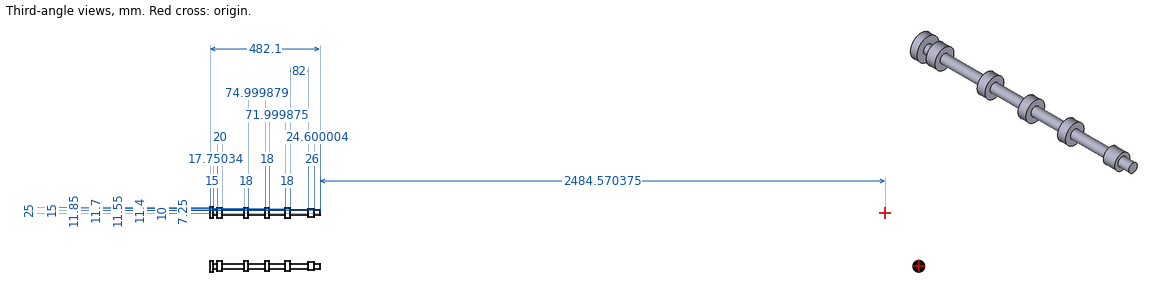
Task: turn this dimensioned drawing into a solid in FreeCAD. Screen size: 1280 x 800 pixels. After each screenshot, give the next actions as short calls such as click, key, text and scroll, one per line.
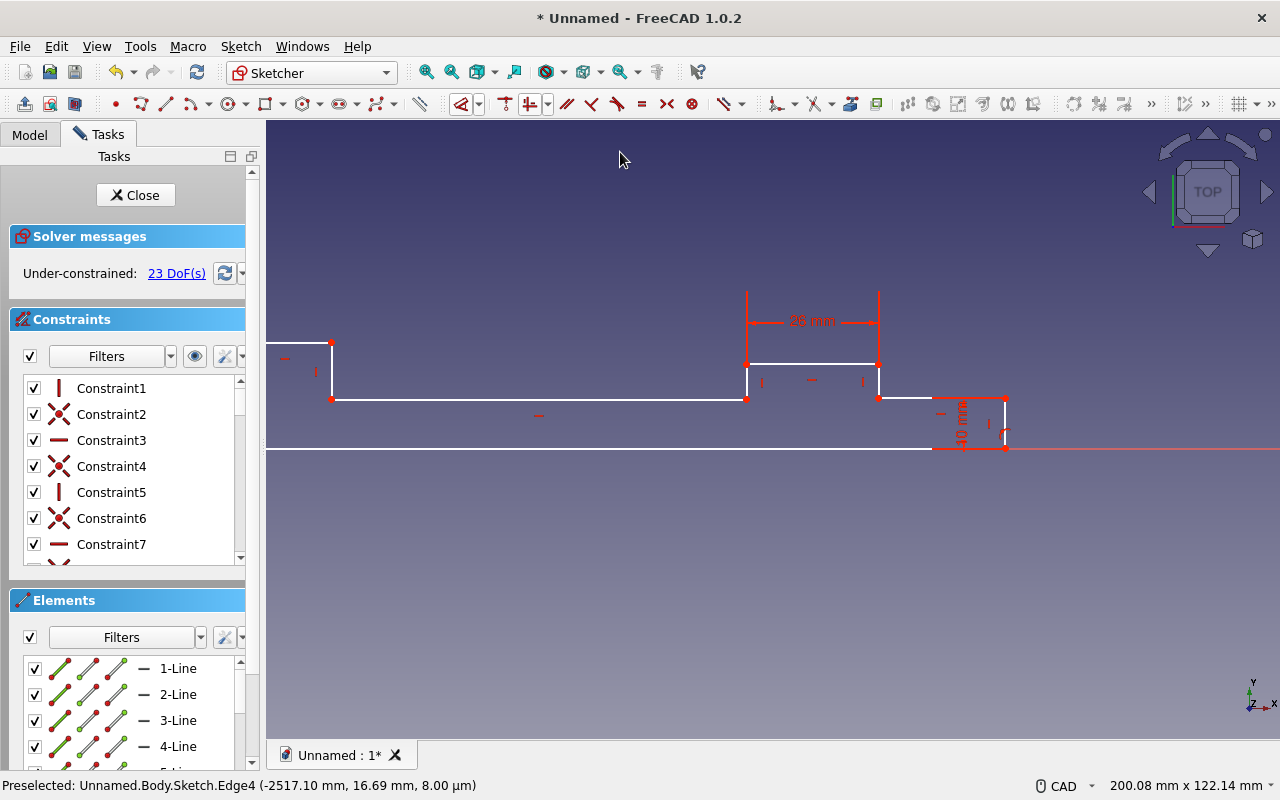
scroll(1006, 444, down, 7)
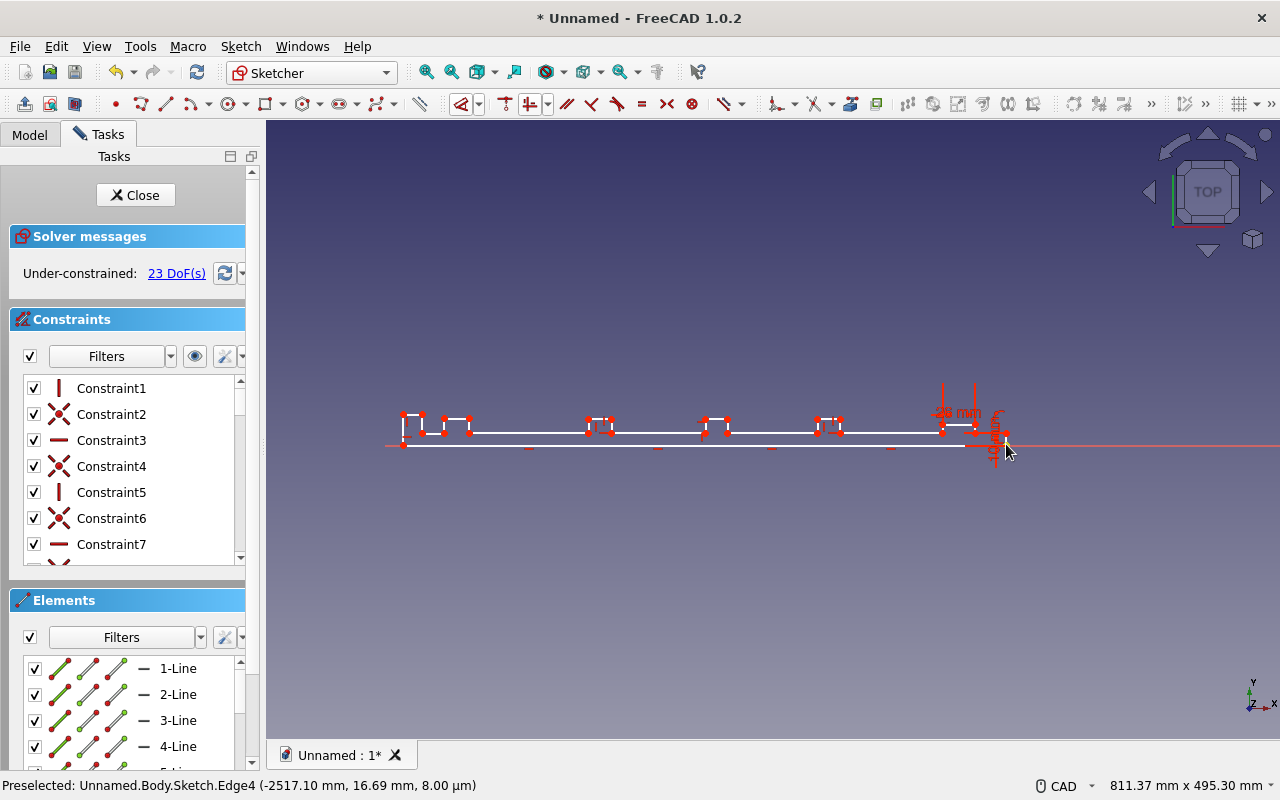
click(912, 433)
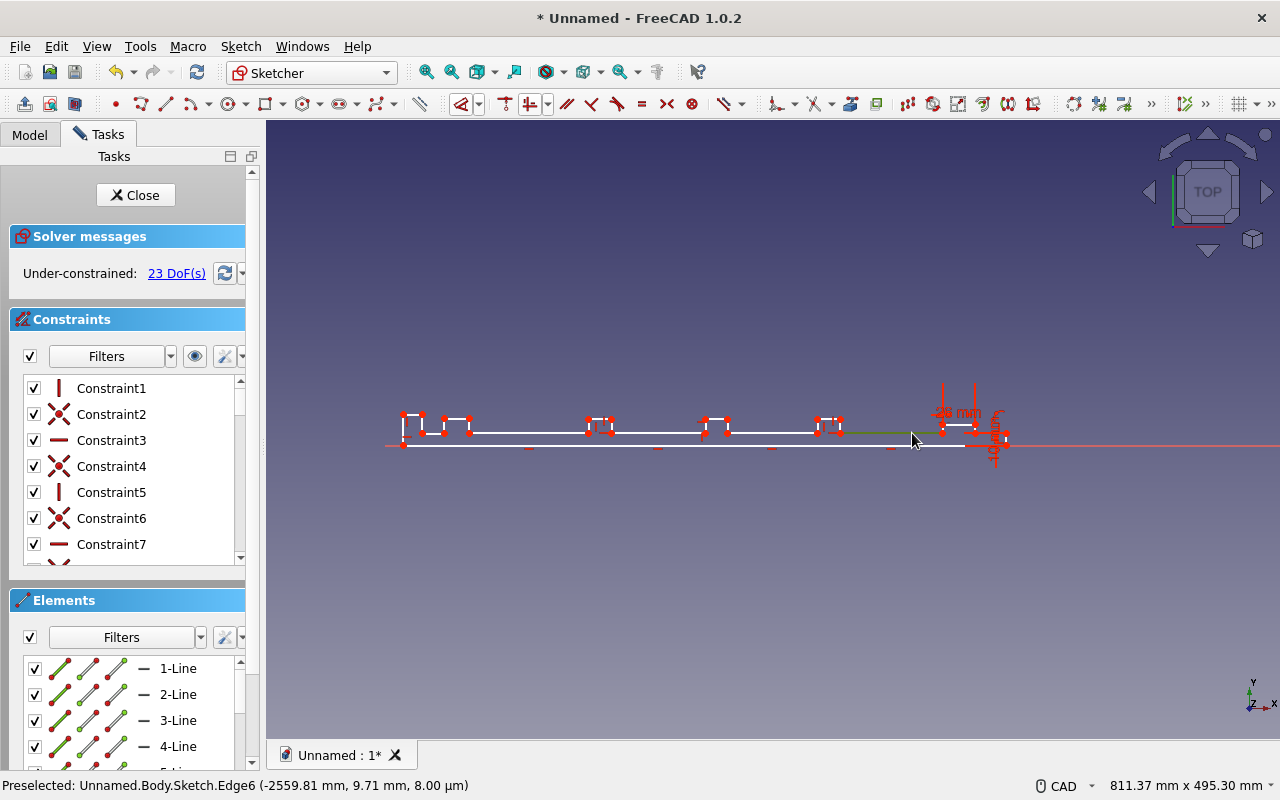
click(478, 104)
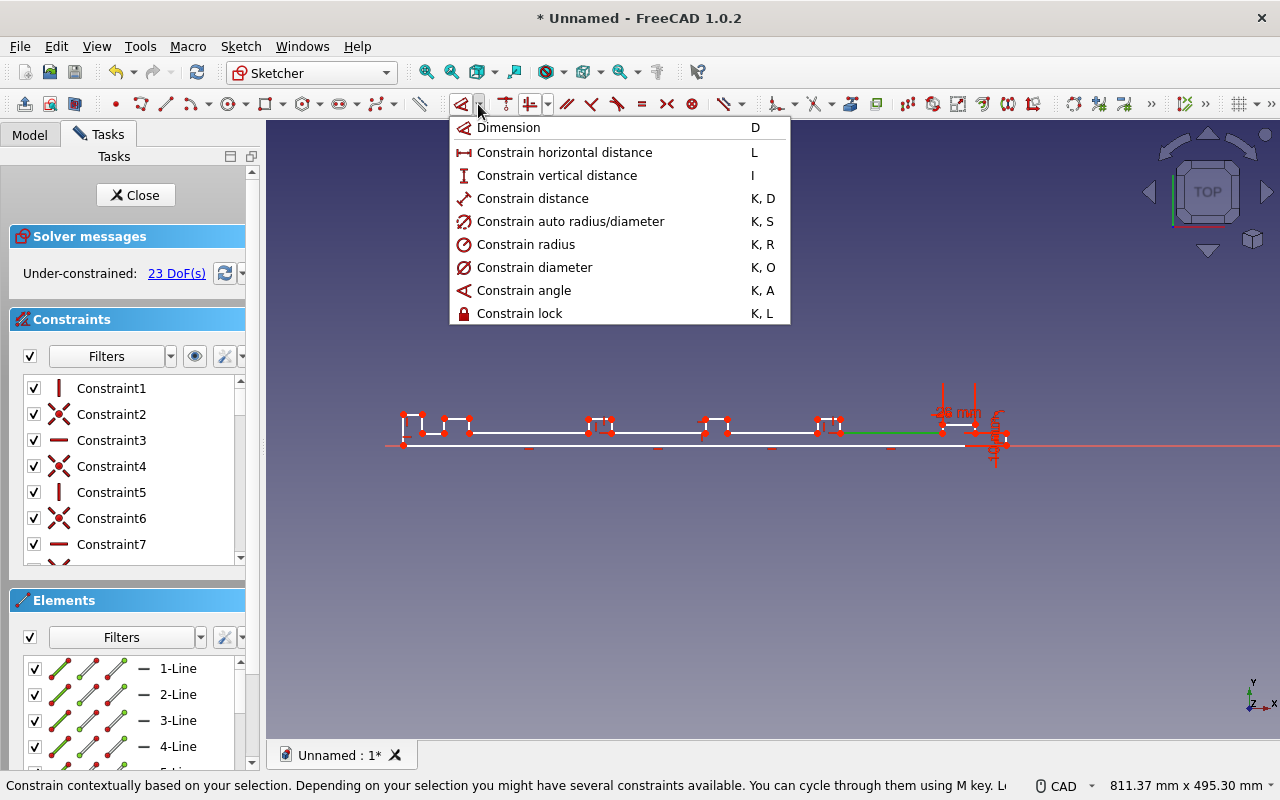
click(620, 152)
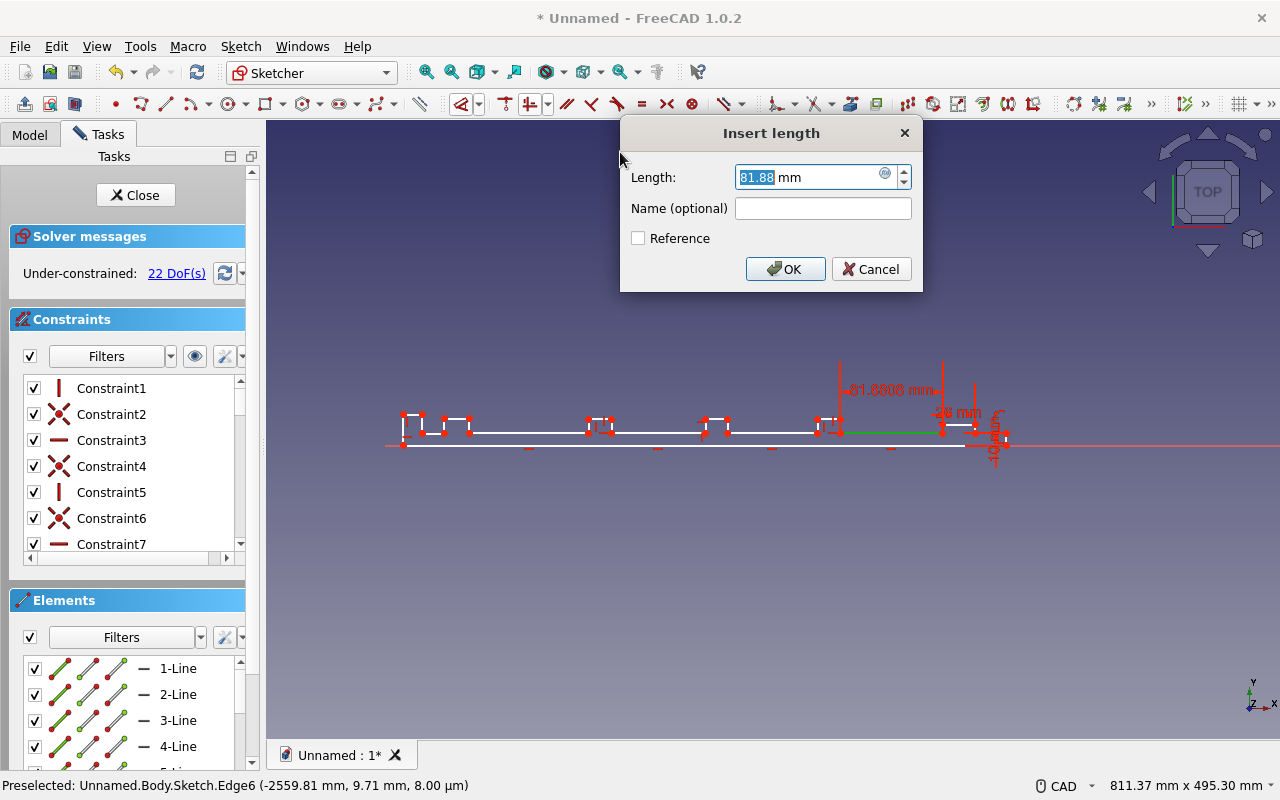
text(82)
key(Return)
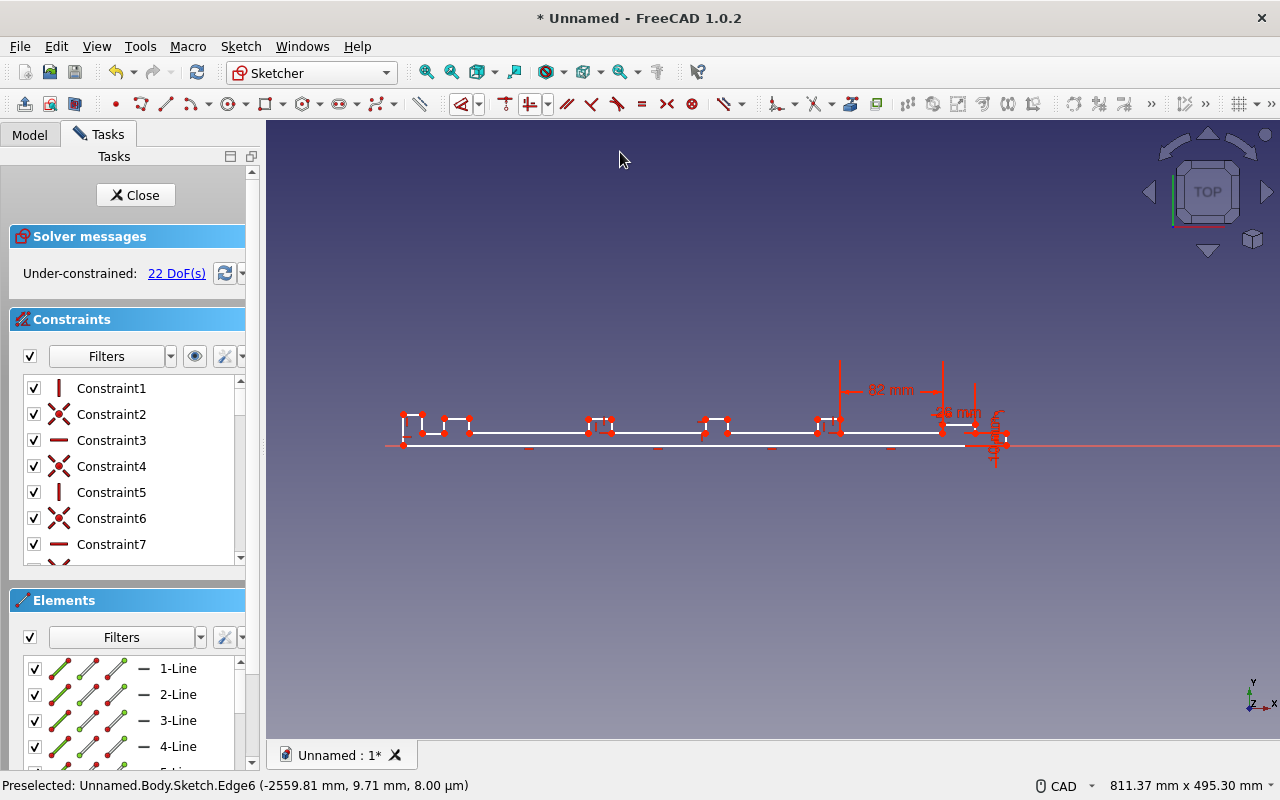
scroll(831, 419, up, 3)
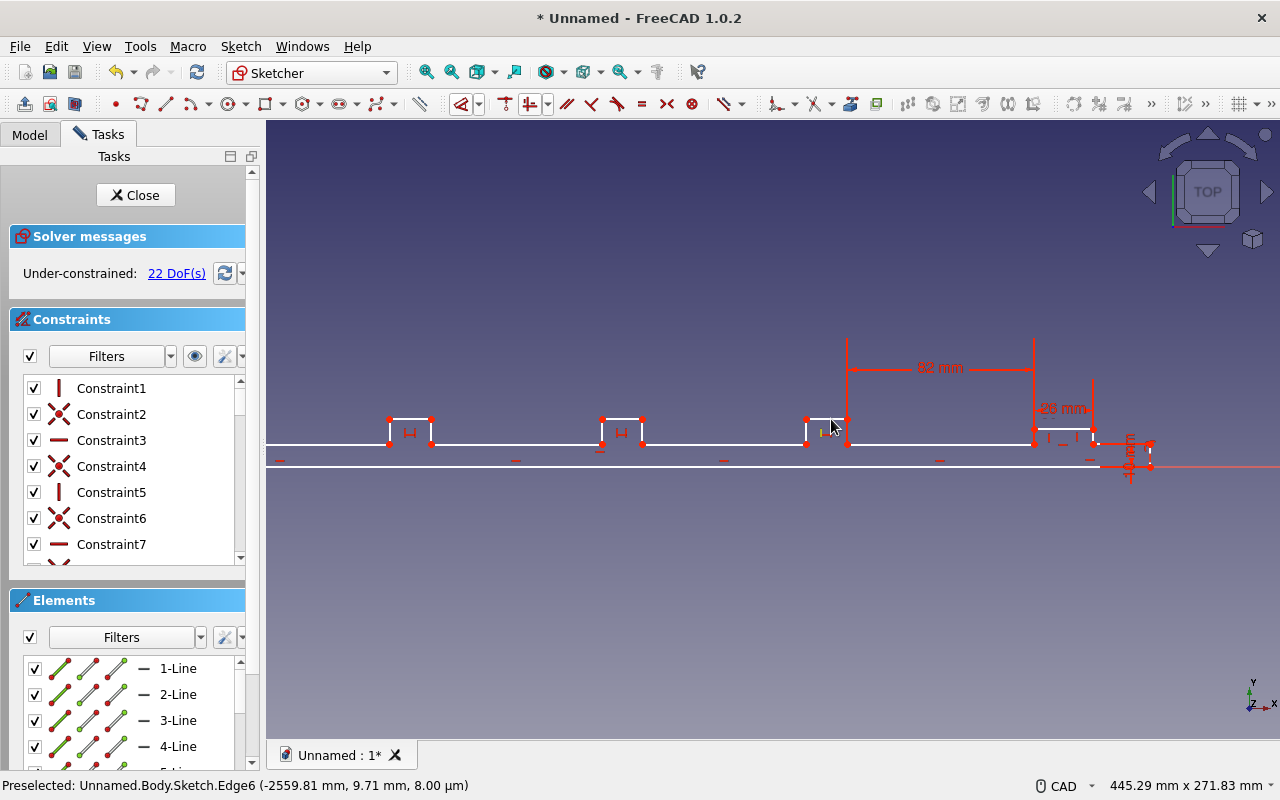
click(831, 419)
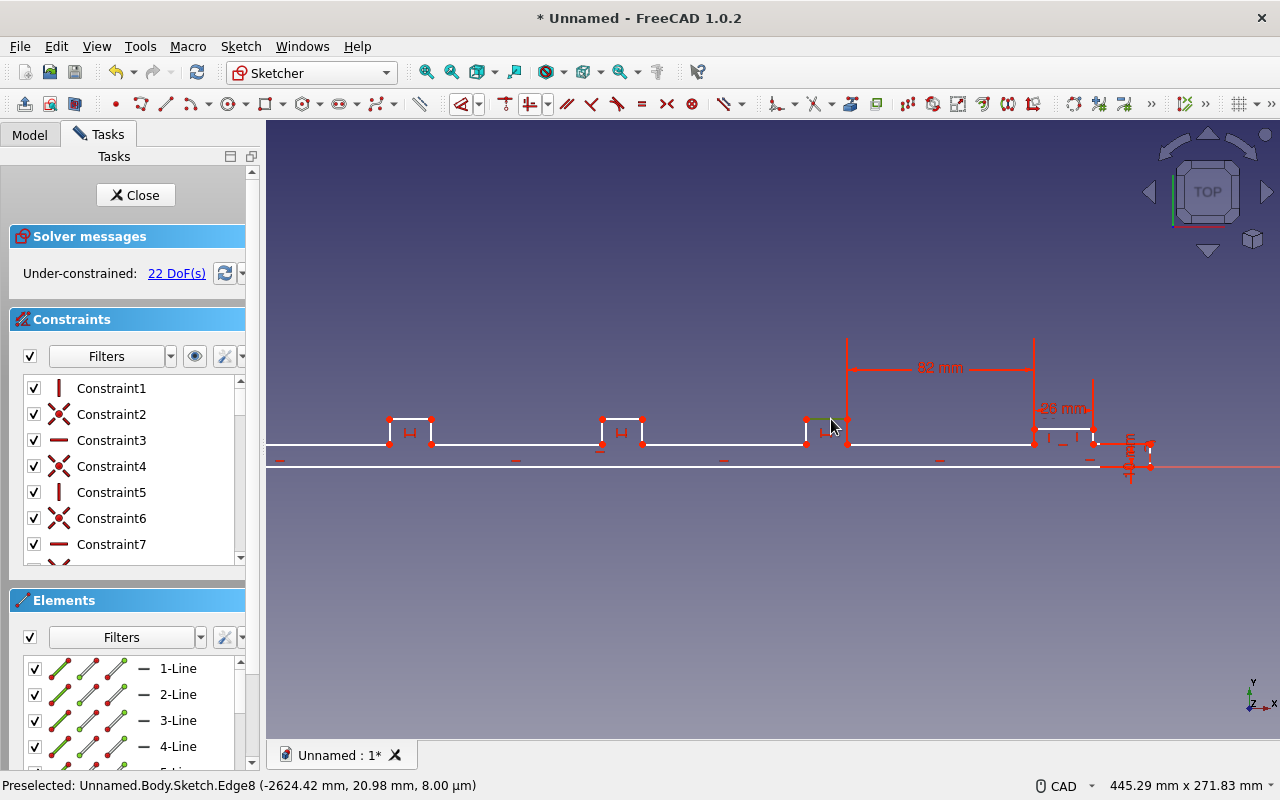
click(478, 104)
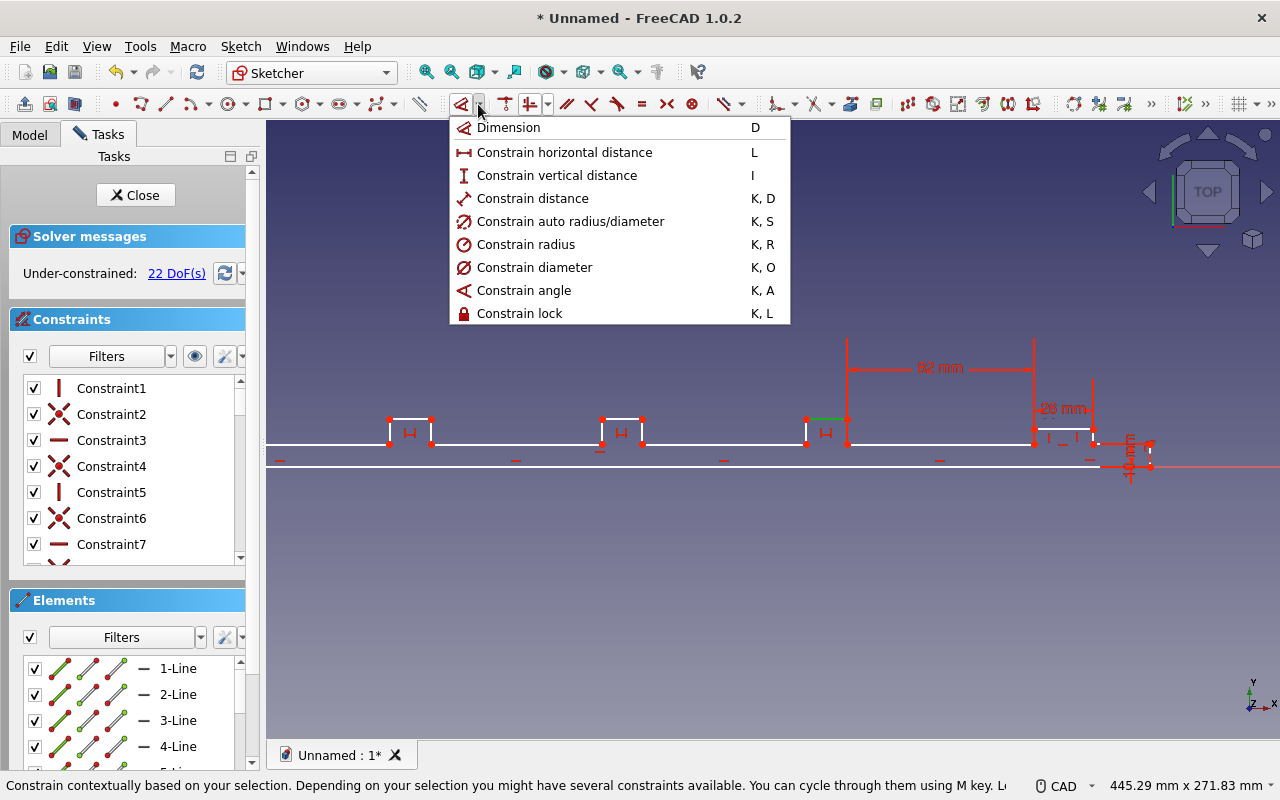
click(620, 152)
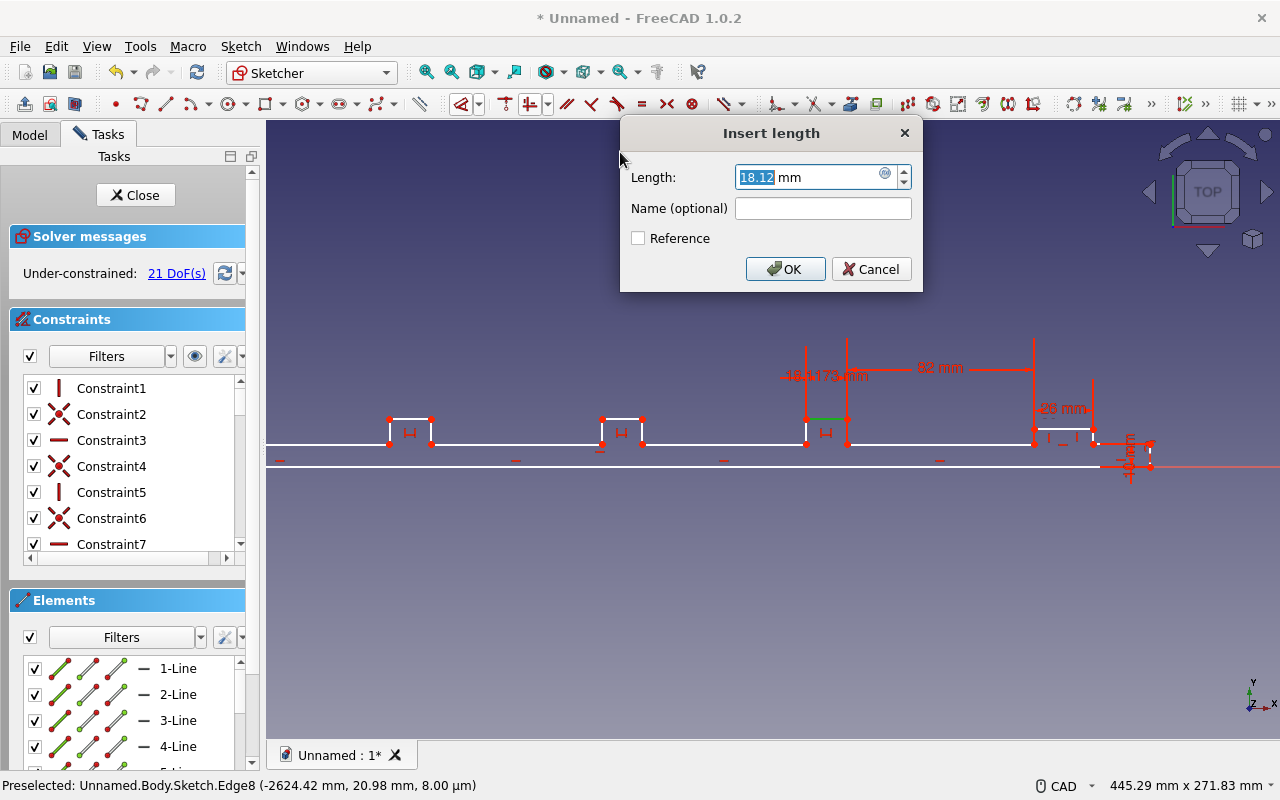
text(18)
key(Return)